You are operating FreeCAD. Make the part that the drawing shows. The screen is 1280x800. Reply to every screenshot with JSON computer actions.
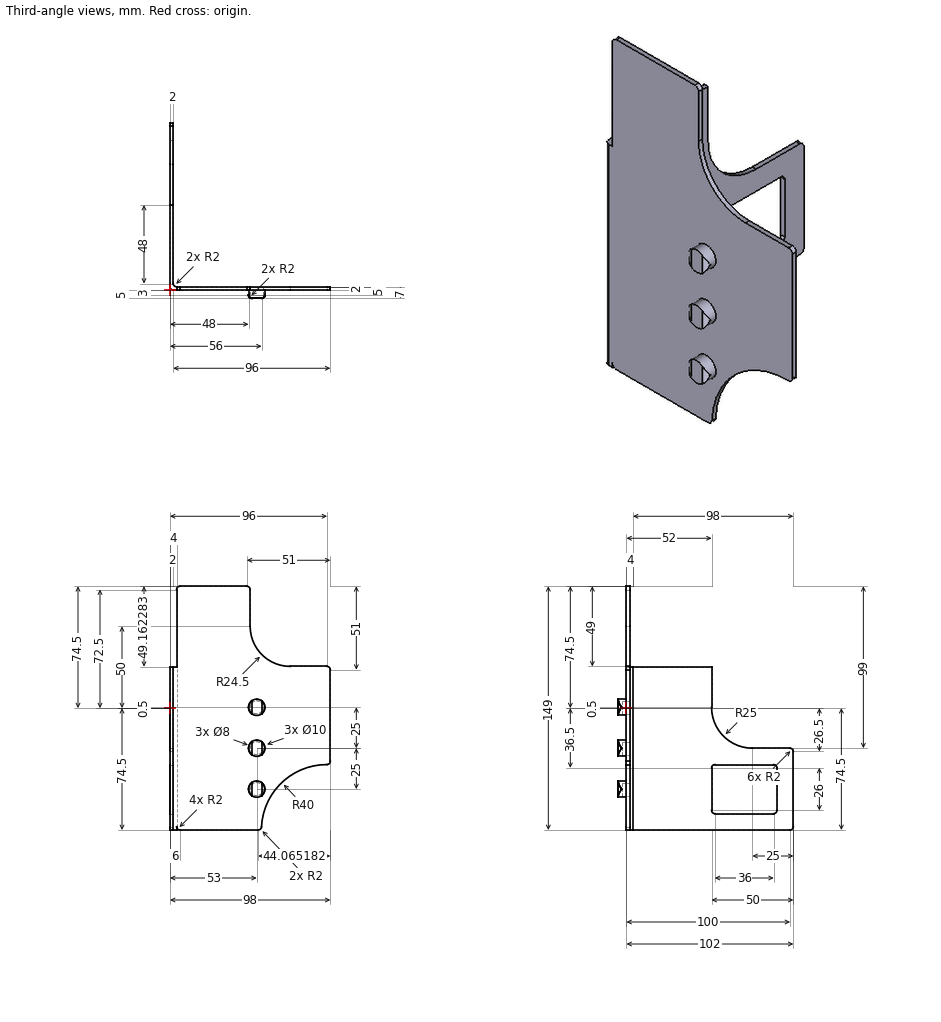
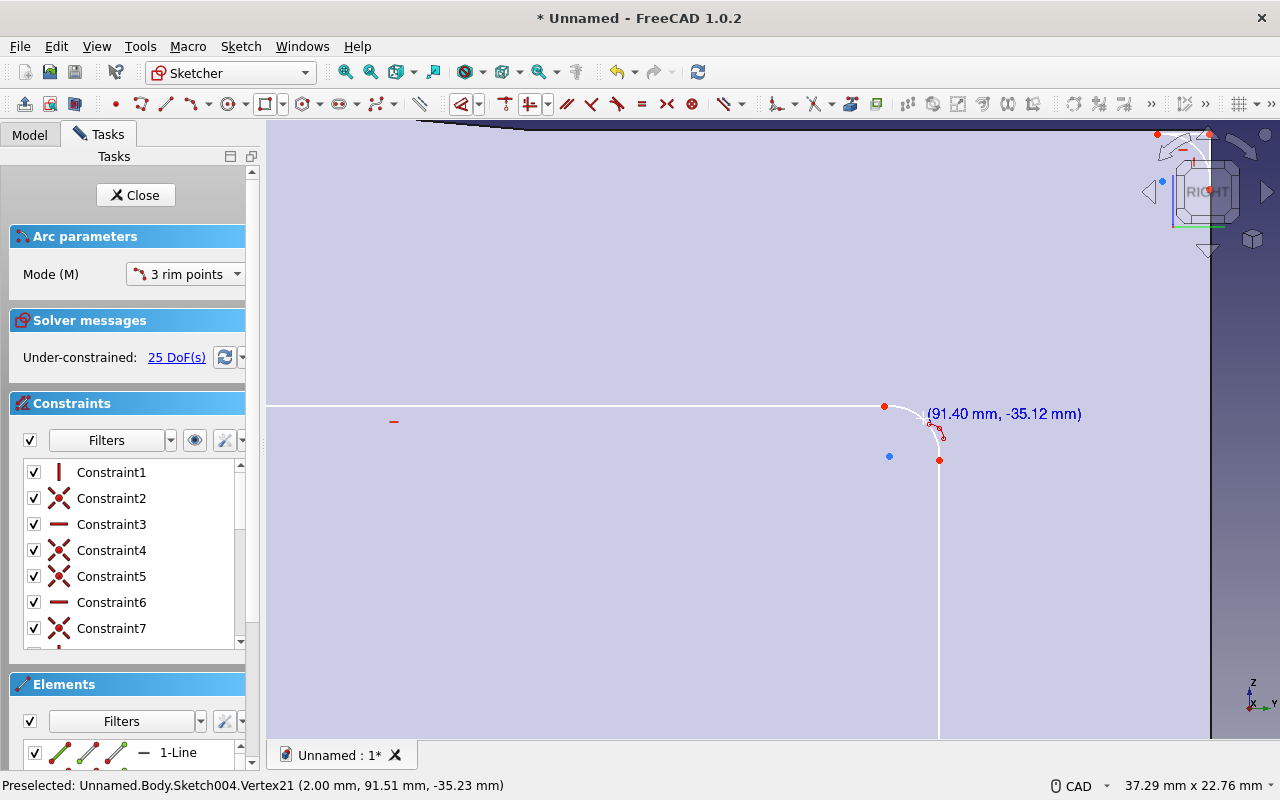
{"action": "scroll", "coordinate": [927, 418], "scroll_direction": "down", "scroll_amount": 8}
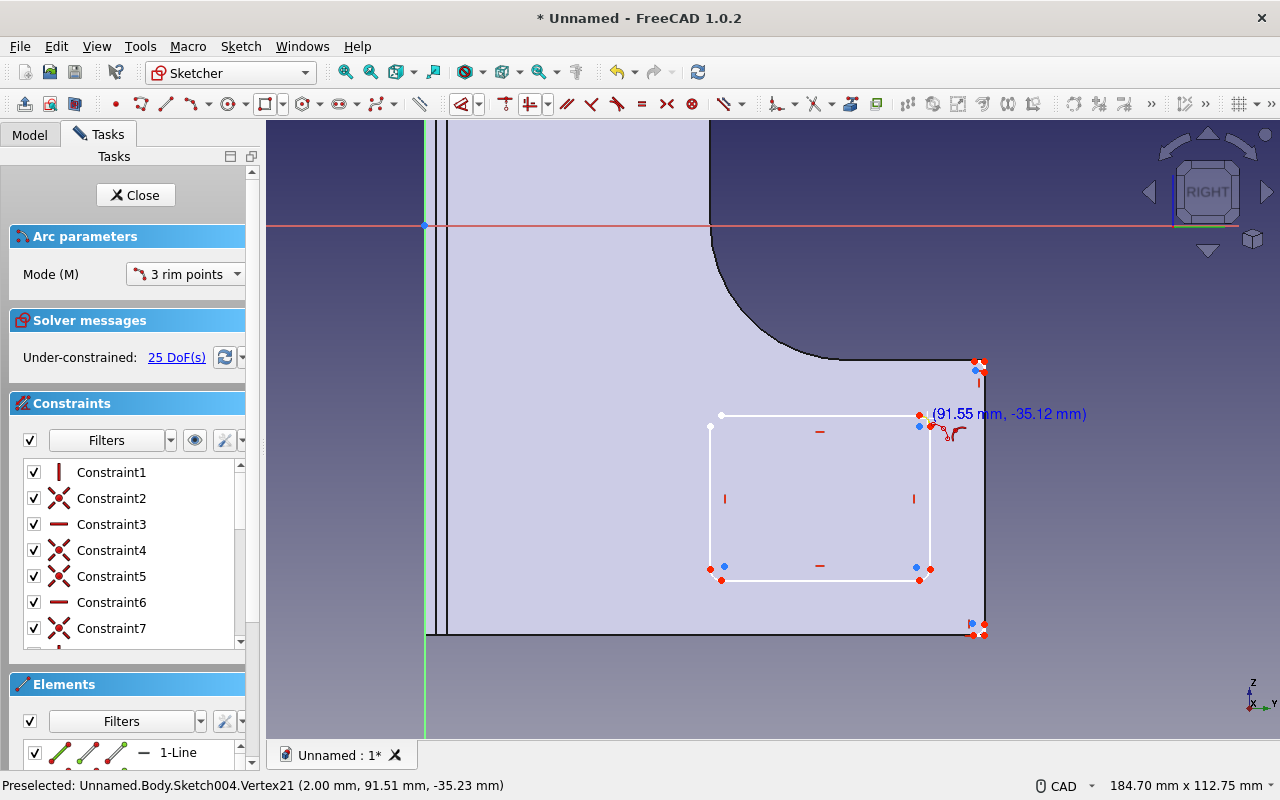
{"action": "left_click", "coordinate": [721, 416]}
{"action": "left_click", "coordinate": [710, 427]}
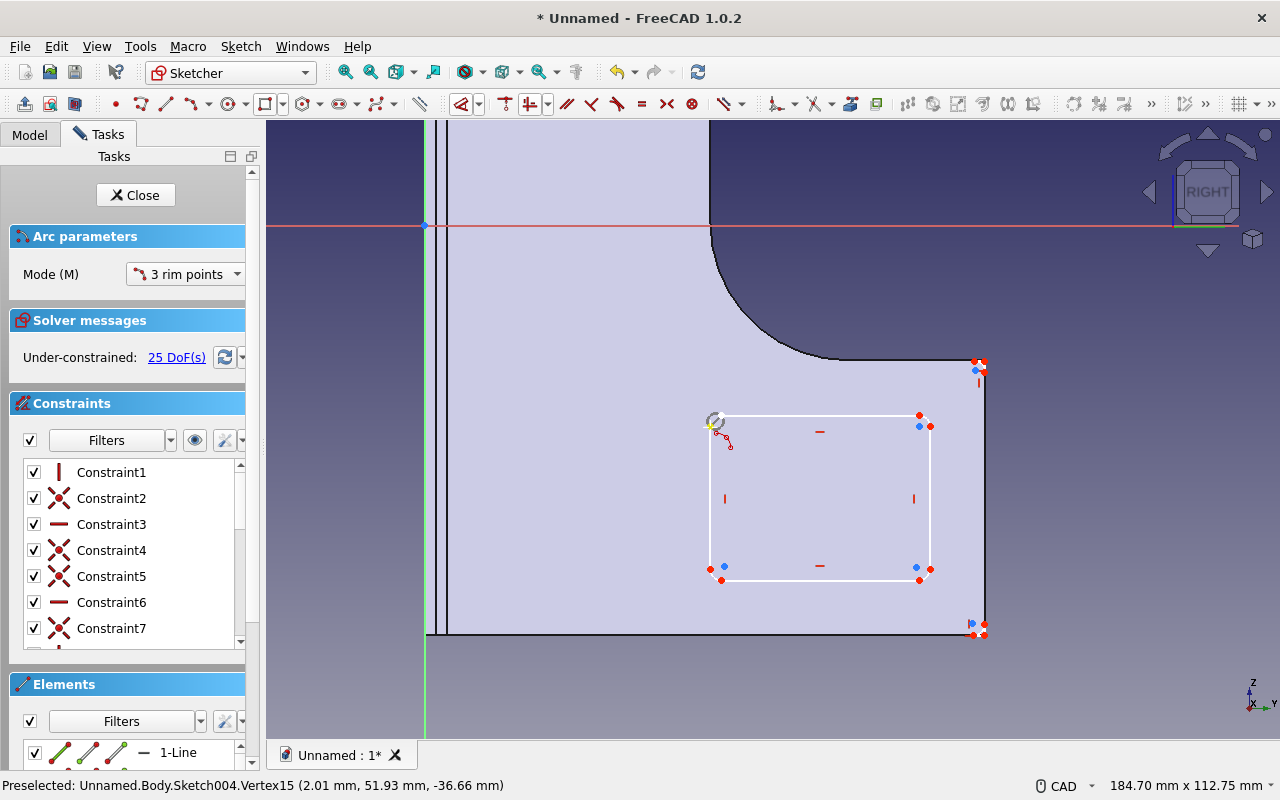
{"action": "scroll", "coordinate": [714, 418], "scroll_direction": "up", "scroll_amount": 8}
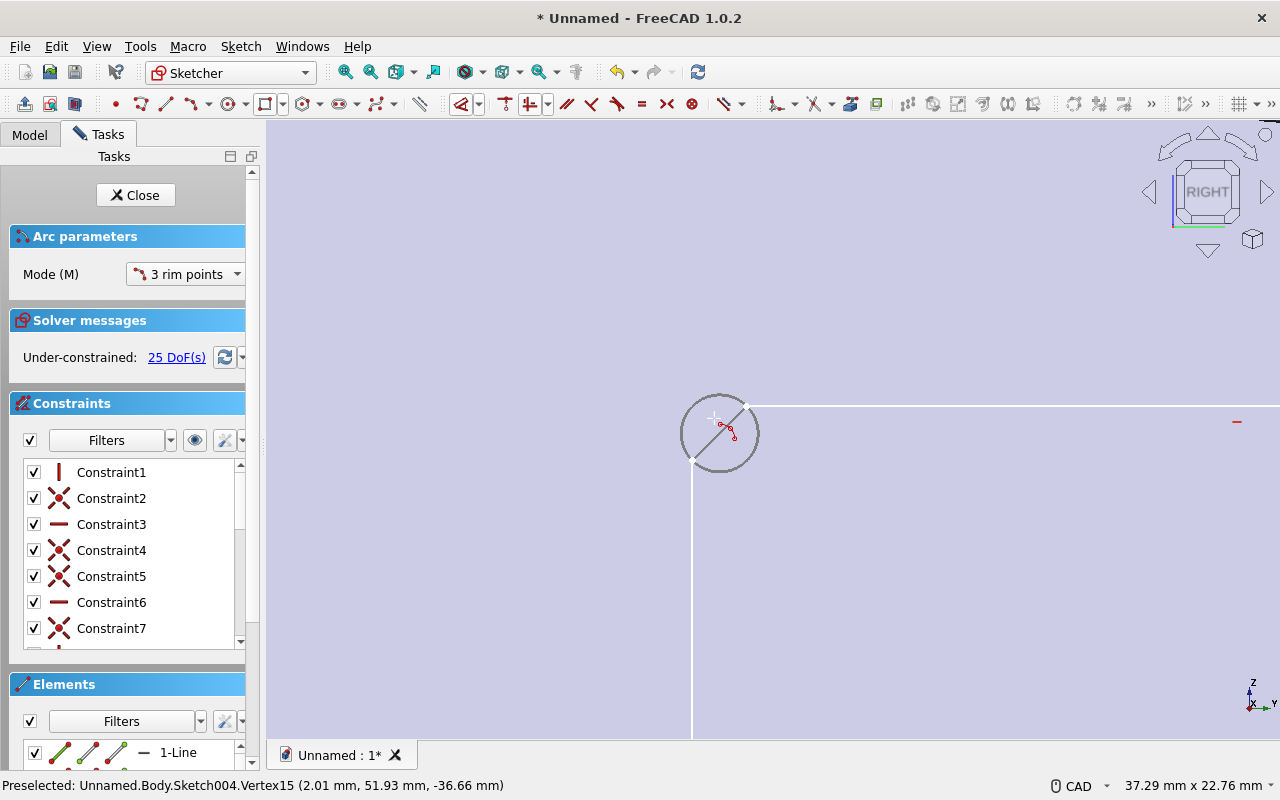
{"action": "left_click", "coordinate": [710, 418]}
{"action": "key", "text": "Escape"}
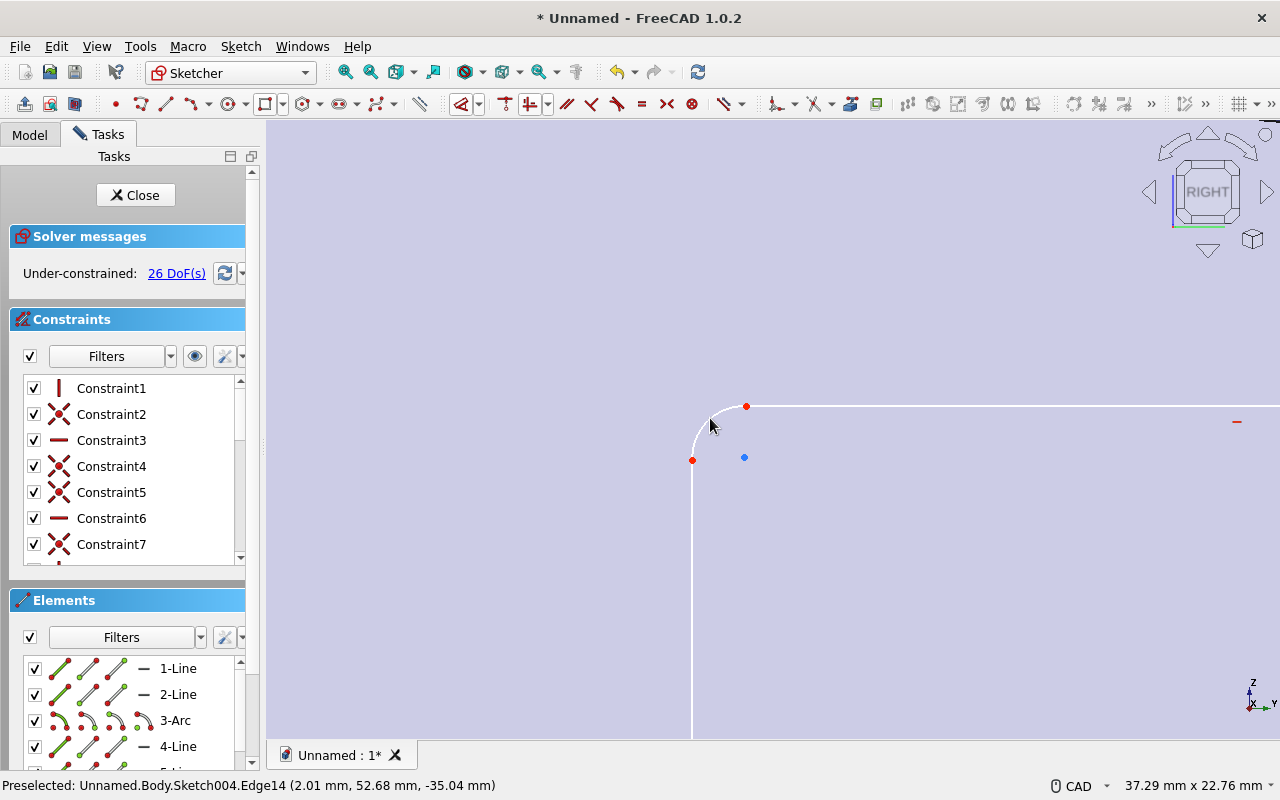
{"action": "scroll", "coordinate": [714, 418], "scroll_direction": "down", "scroll_amount": 8}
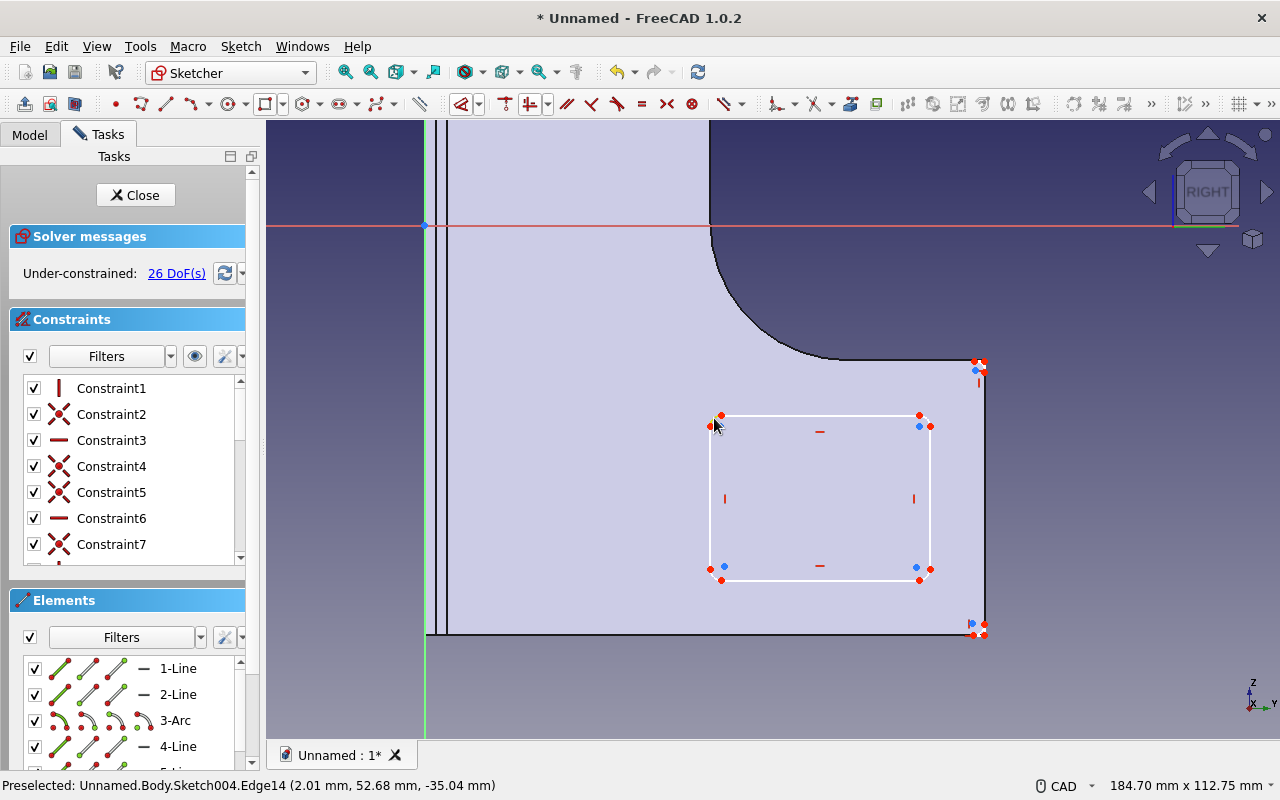
{"action": "scroll", "coordinate": [985, 363], "scroll_direction": "up", "scroll_amount": 10}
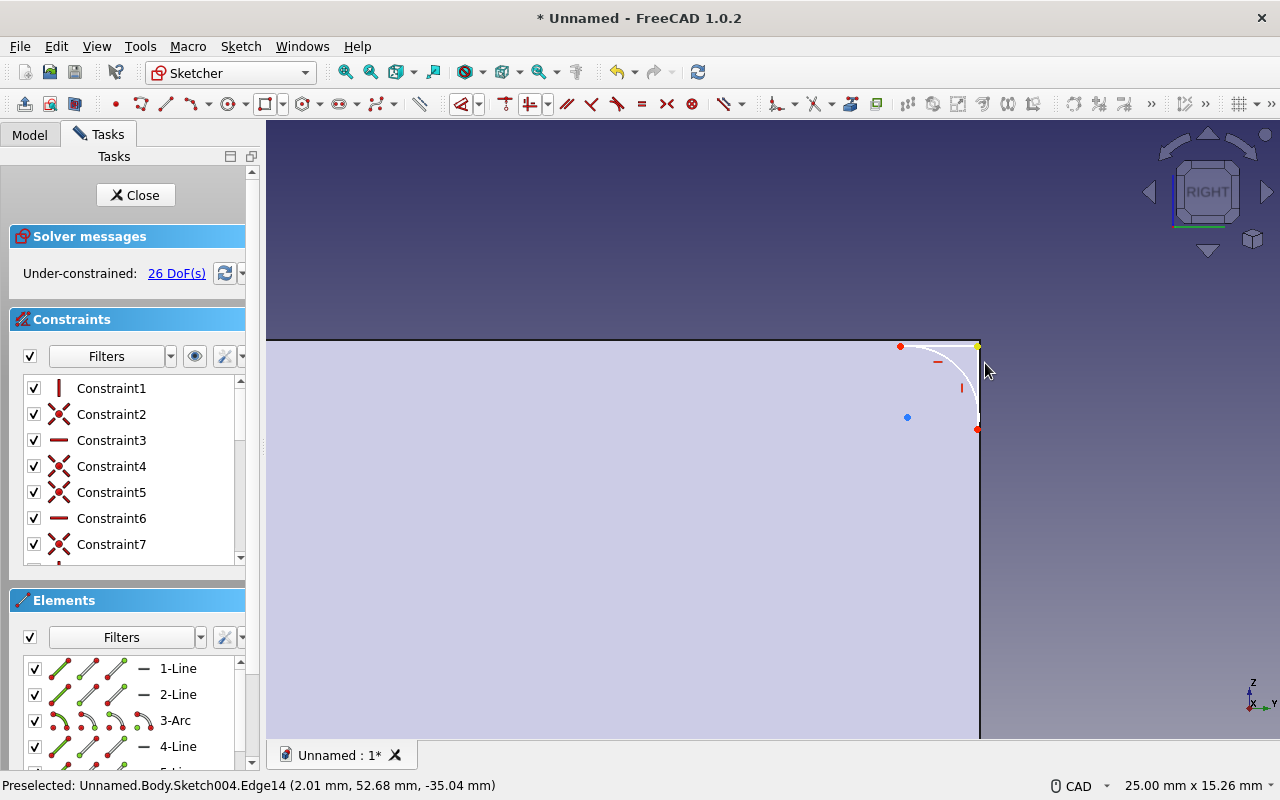
{"action": "left_click", "coordinate": [978, 363]}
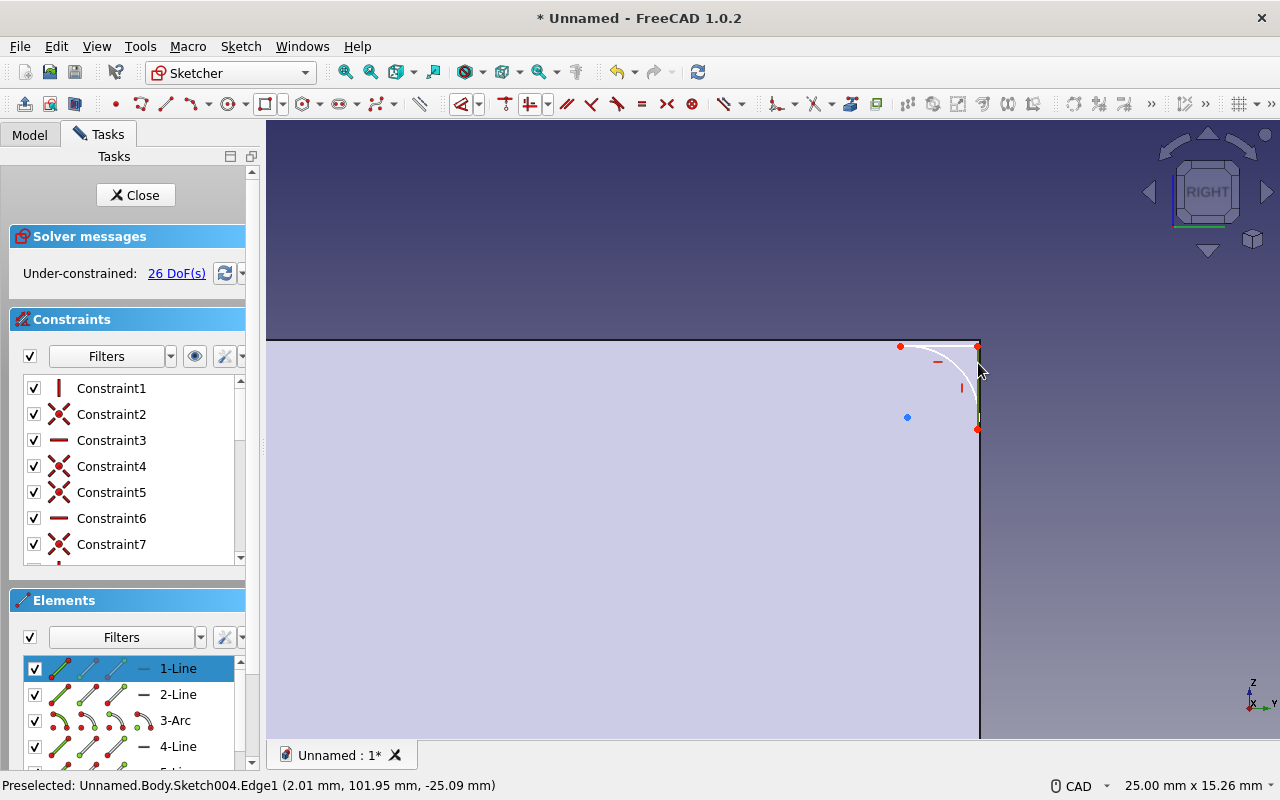
{"action": "left_click", "coordinate": [959, 369]}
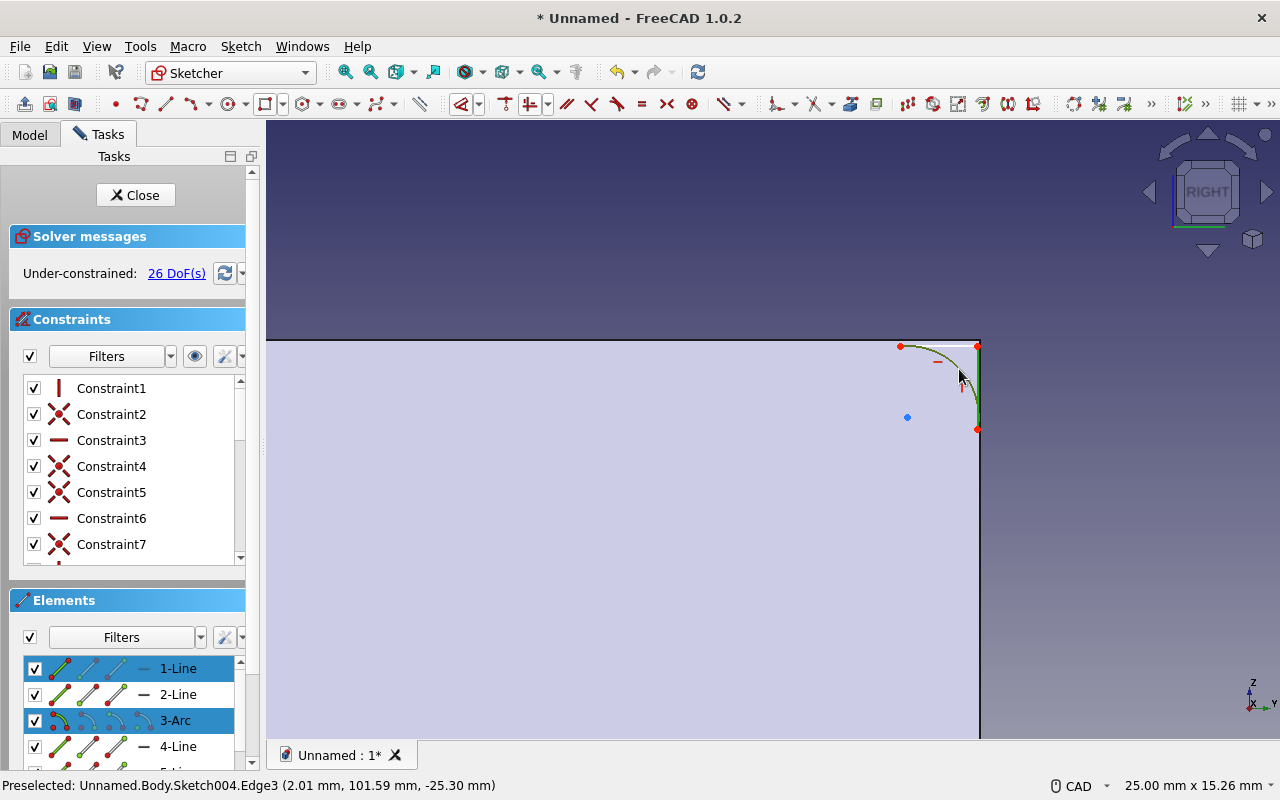
{"action": "key", "text": "t"}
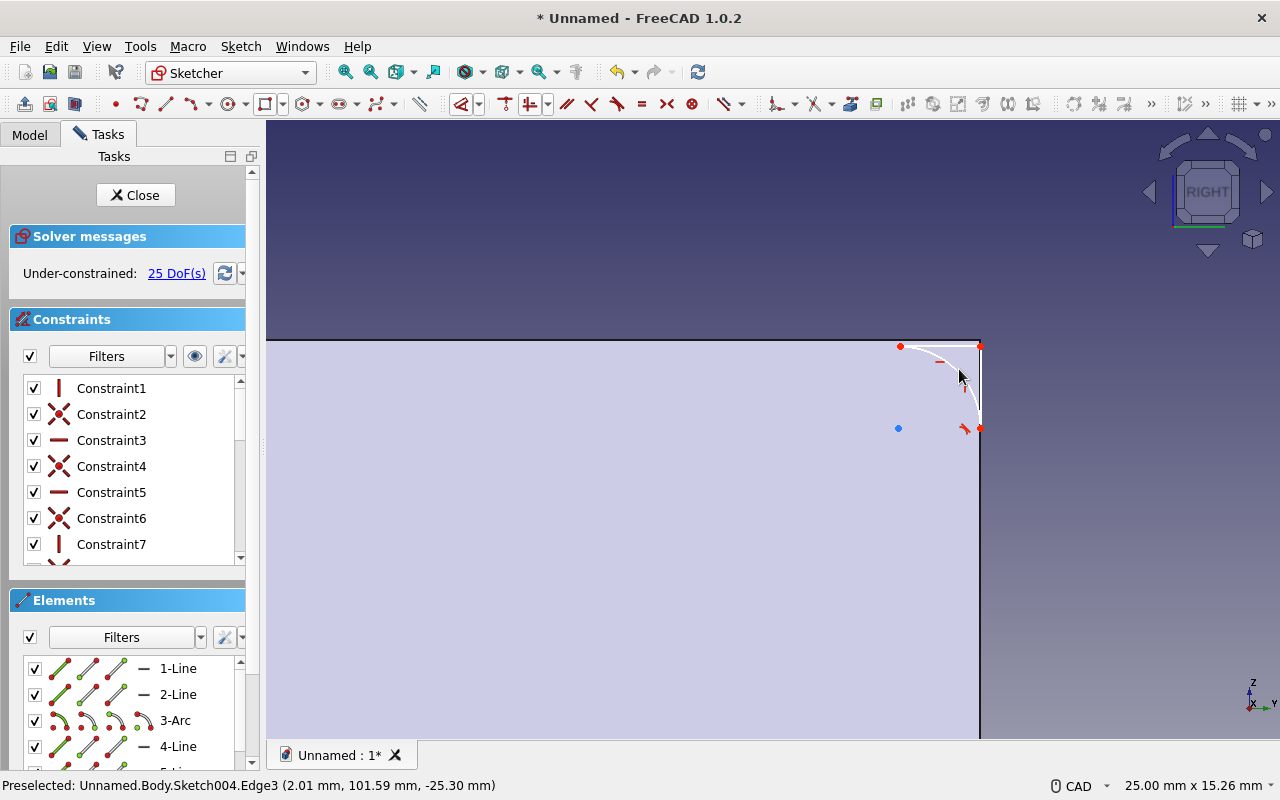
{"action": "left_click", "coordinate": [956, 346]}